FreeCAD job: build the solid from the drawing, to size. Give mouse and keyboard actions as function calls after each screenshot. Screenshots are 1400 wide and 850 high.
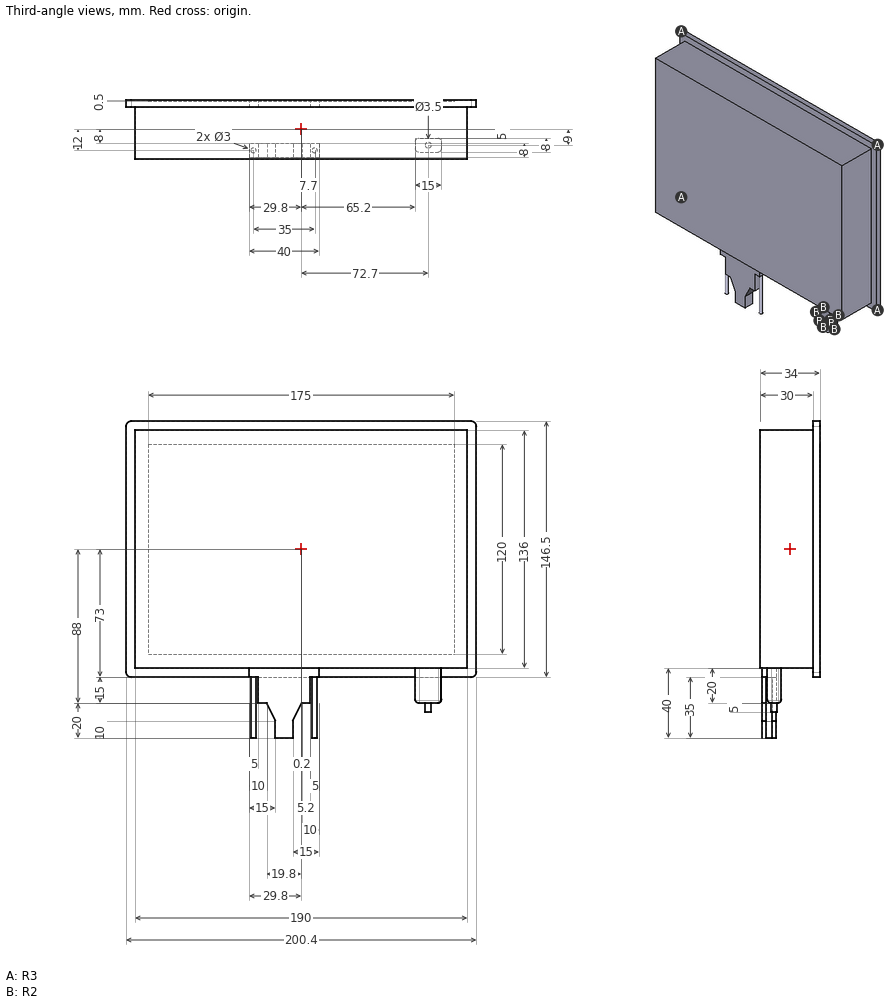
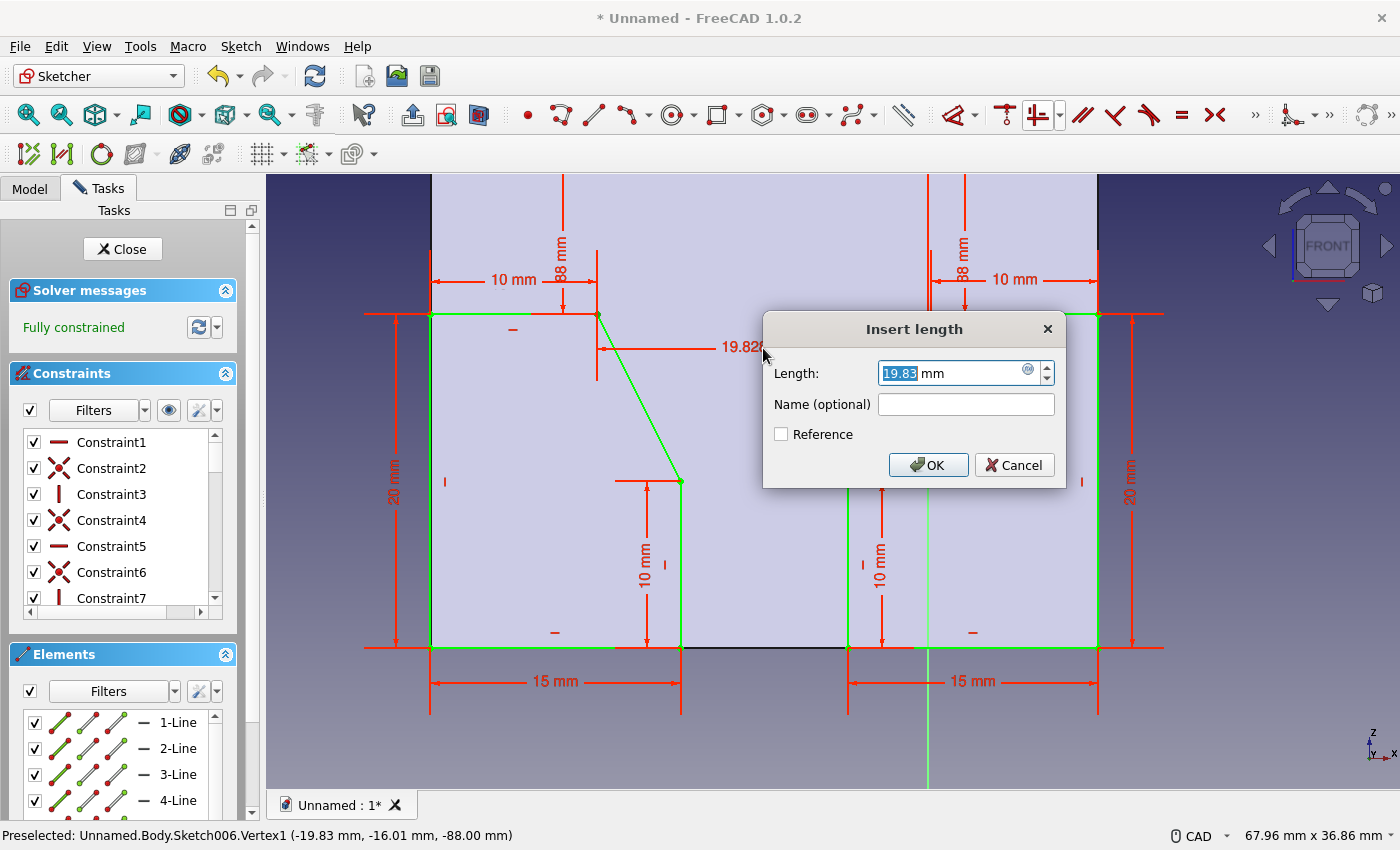
text(19.8)
key(Return)
key(Escape)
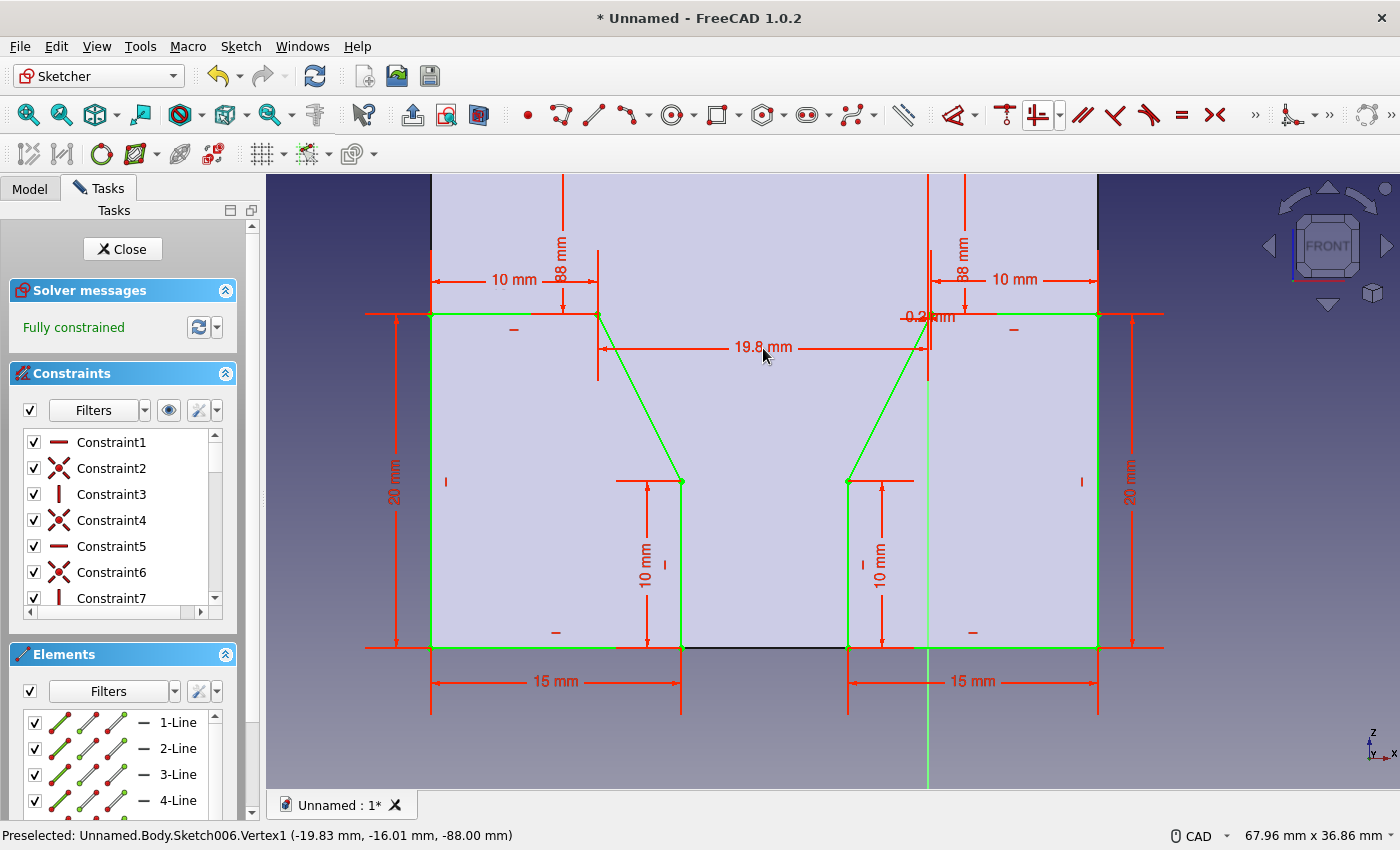
click(123, 249)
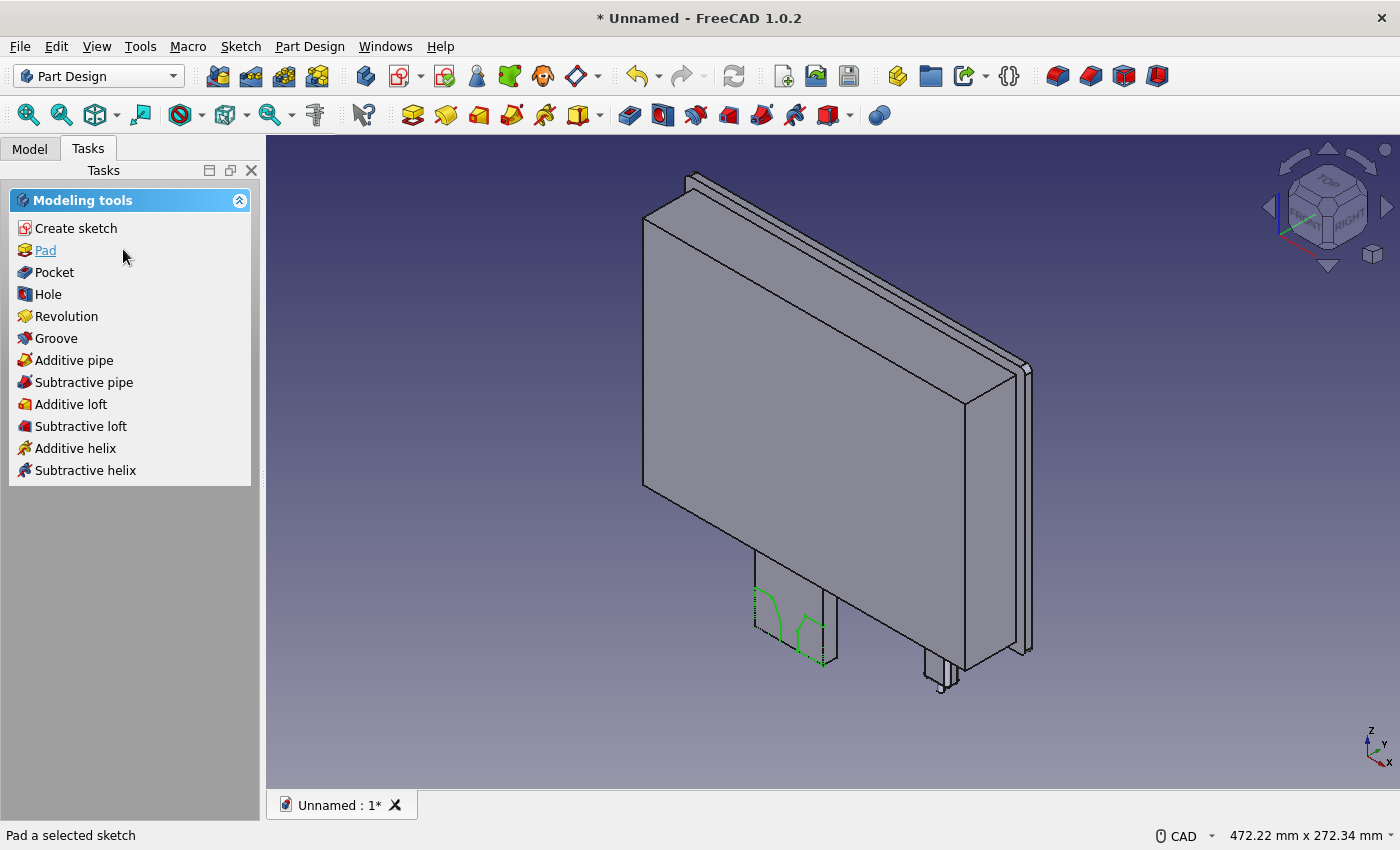
click(630, 116)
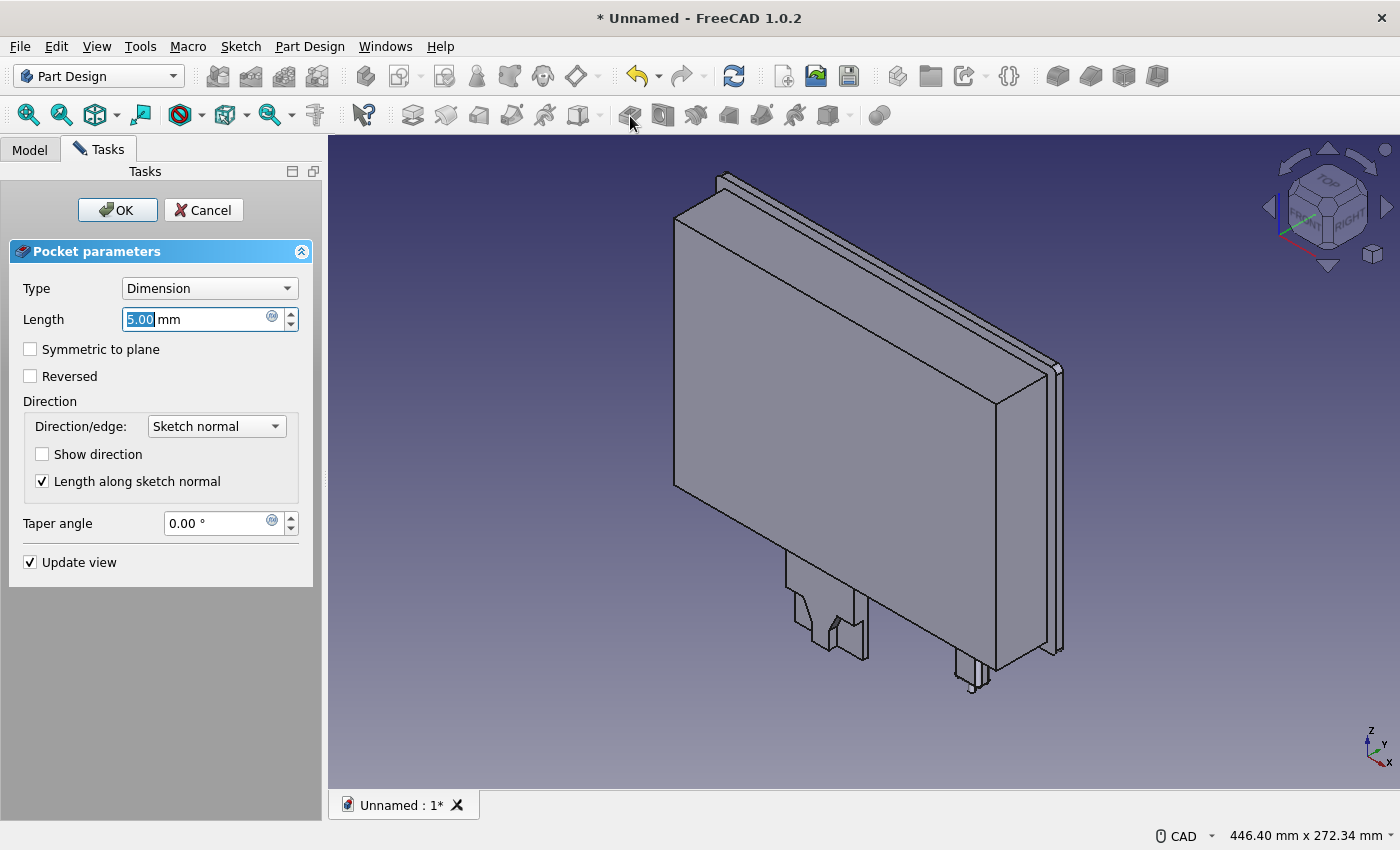
click(210, 288)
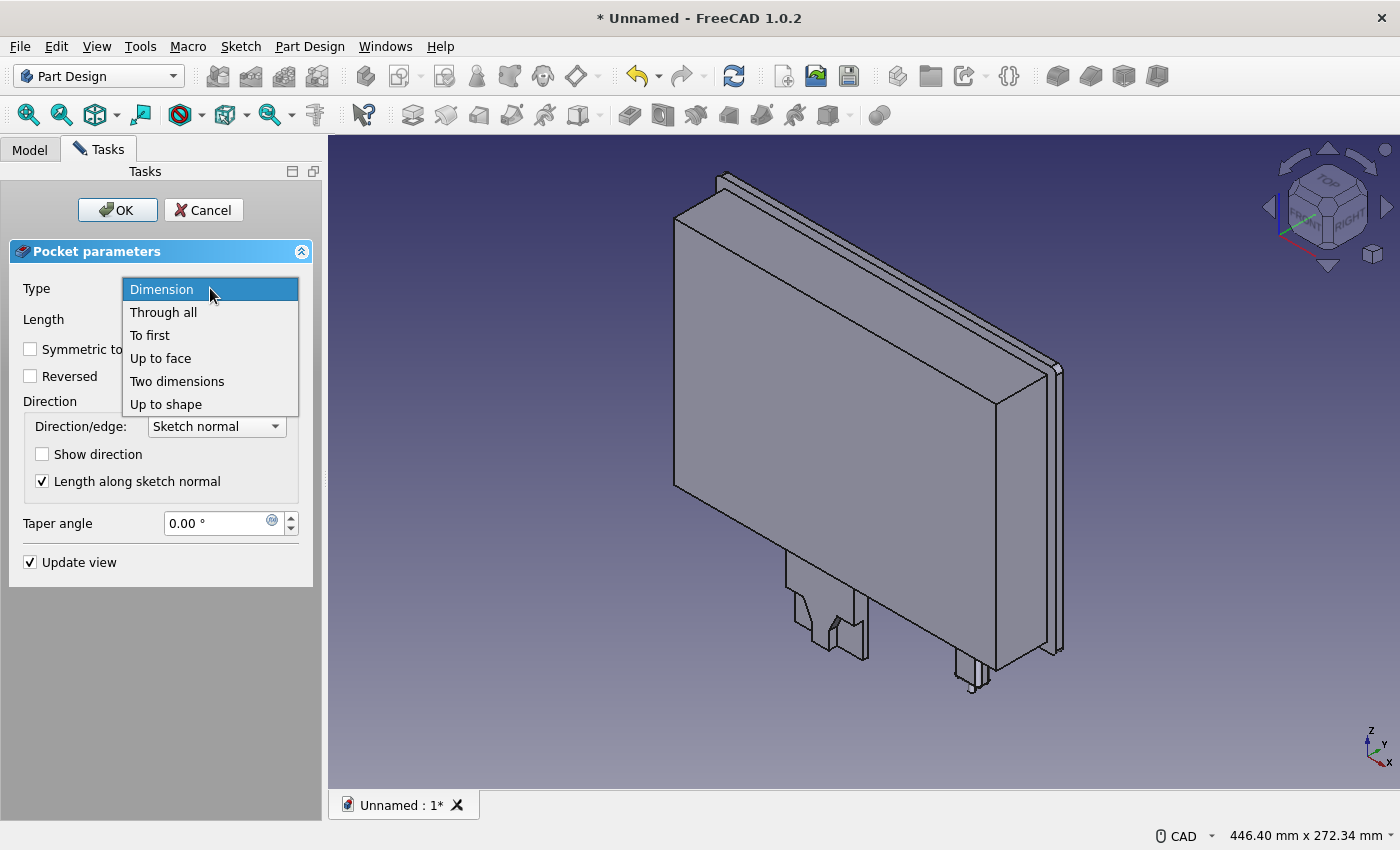
click(208, 312)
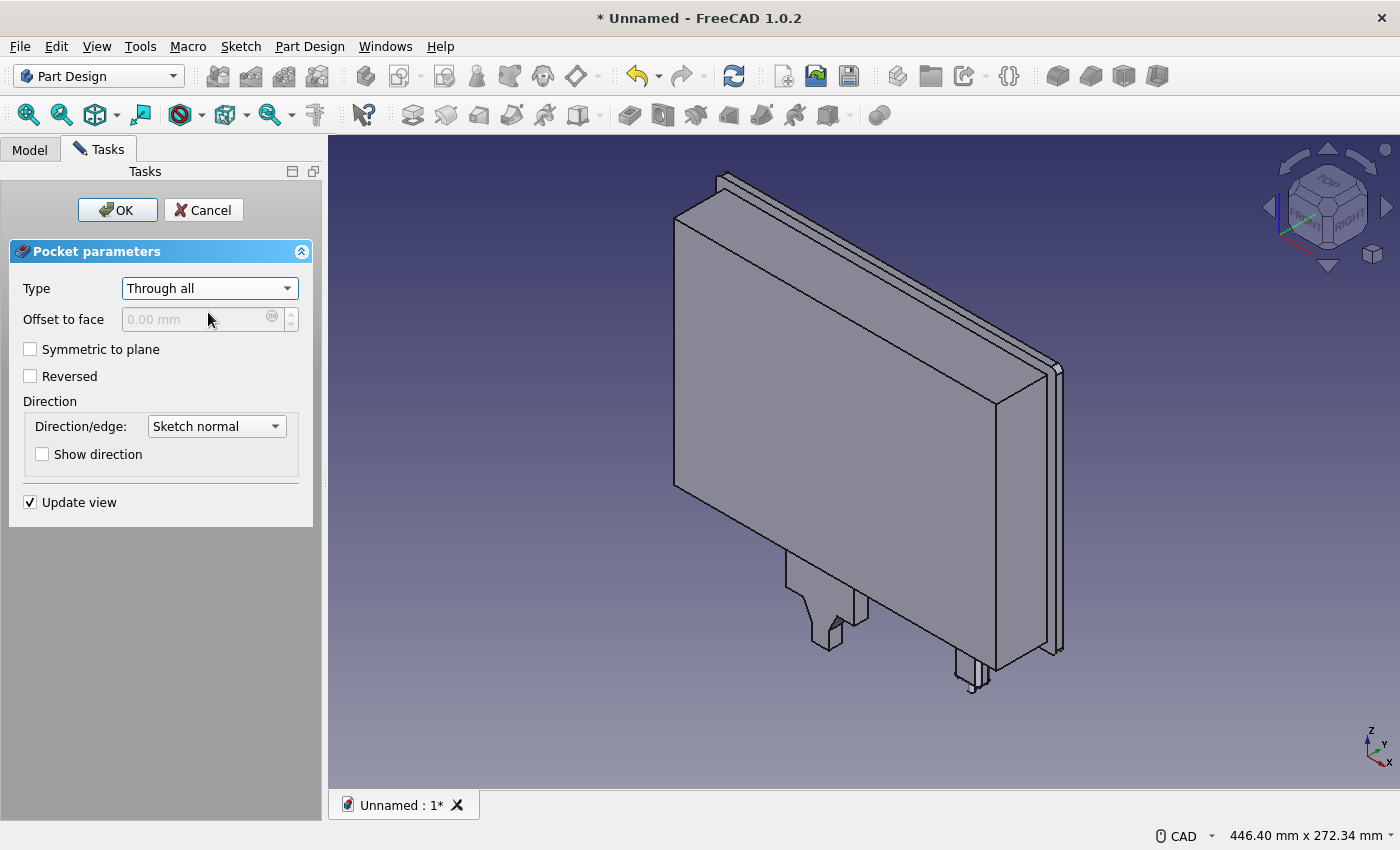
click(118, 210)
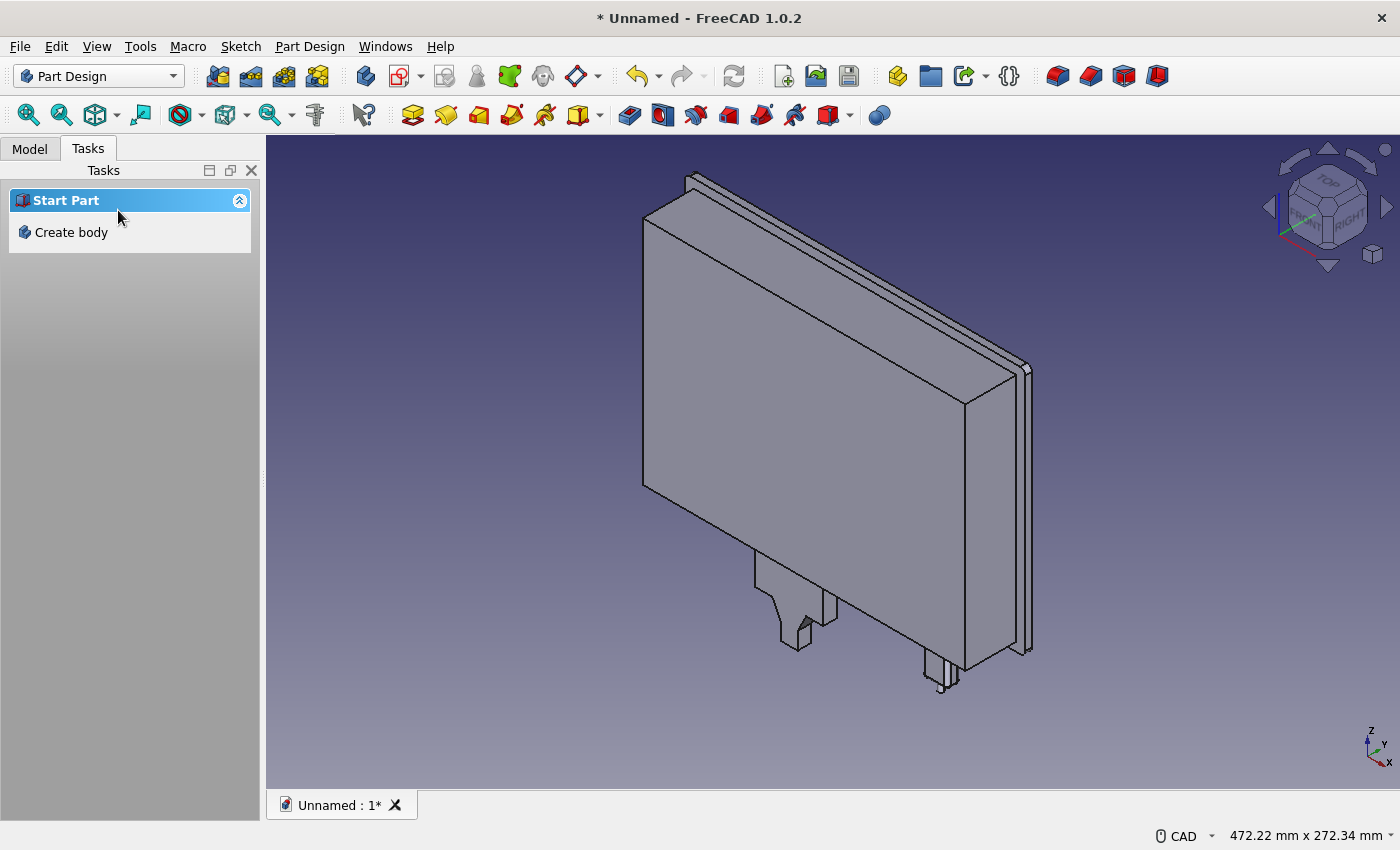
click(789, 594)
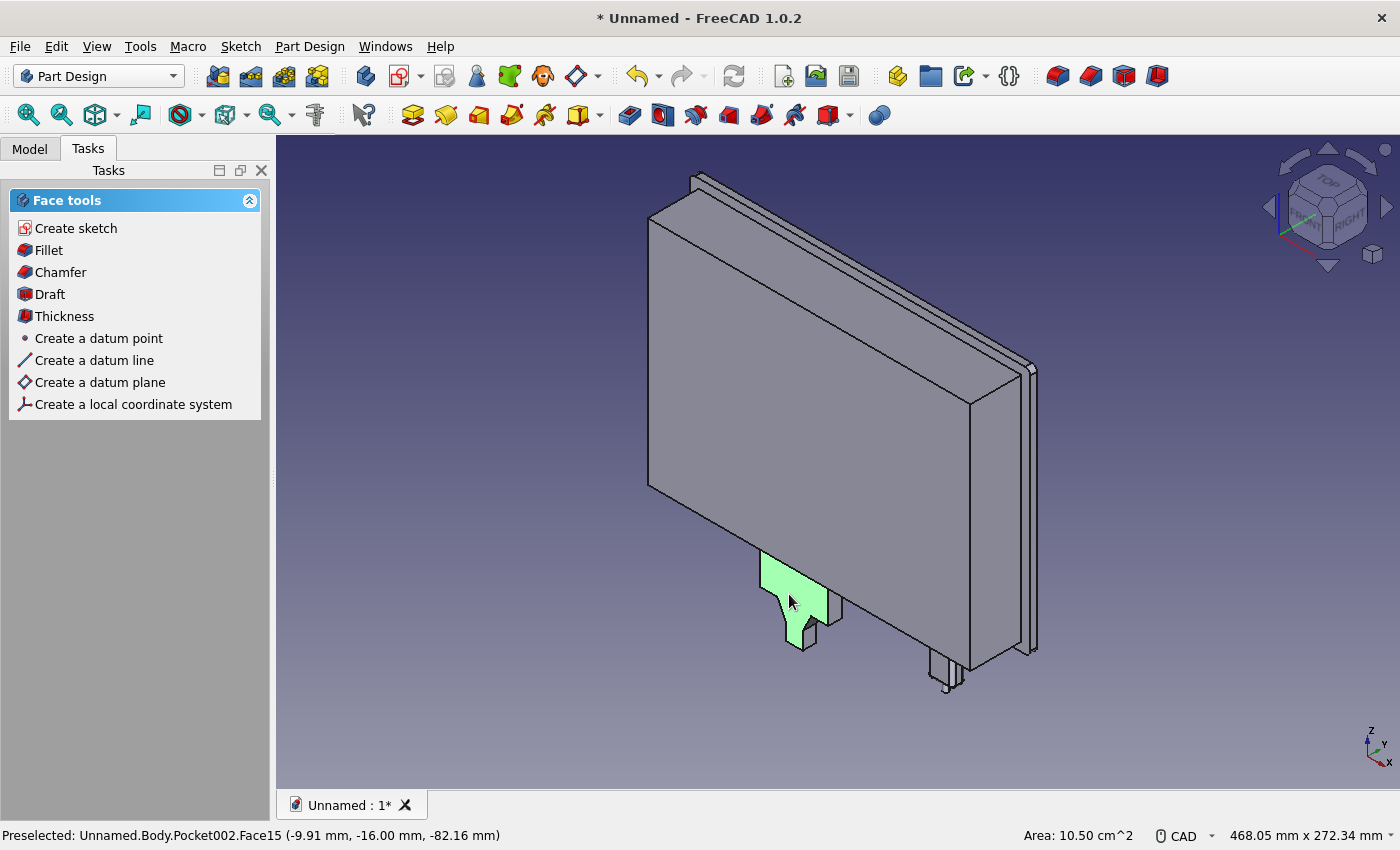
click(398, 76)